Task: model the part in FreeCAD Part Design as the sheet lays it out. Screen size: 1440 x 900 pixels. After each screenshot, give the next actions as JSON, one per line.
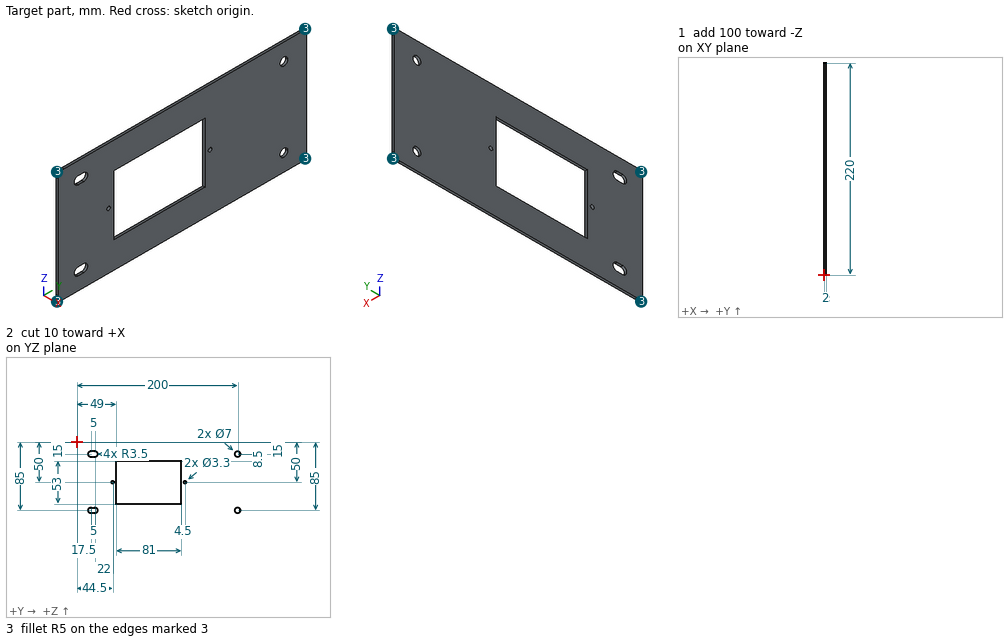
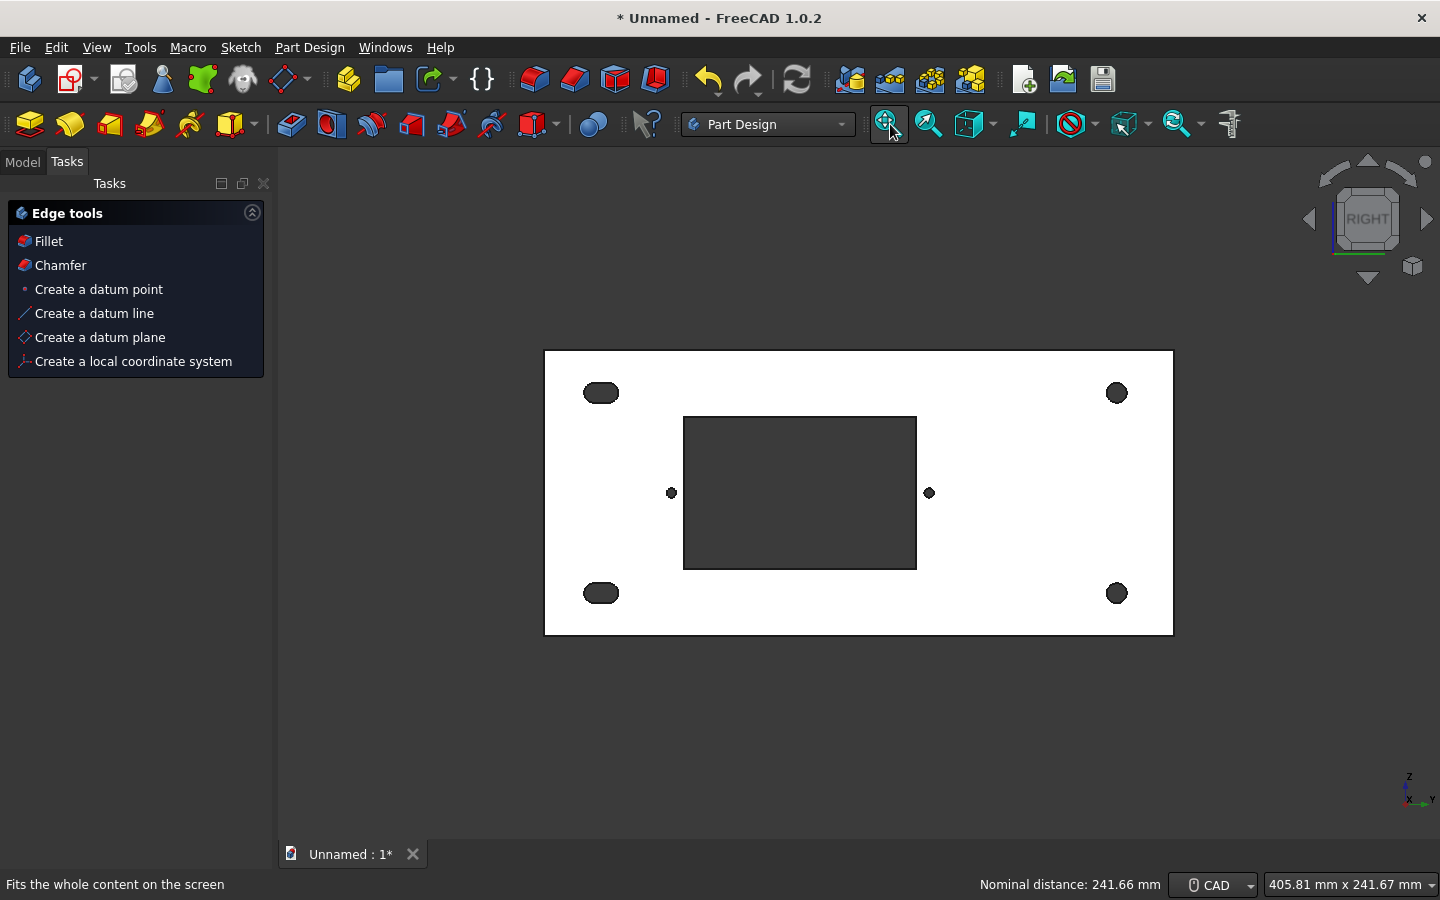
{"action": "key", "text": "5"}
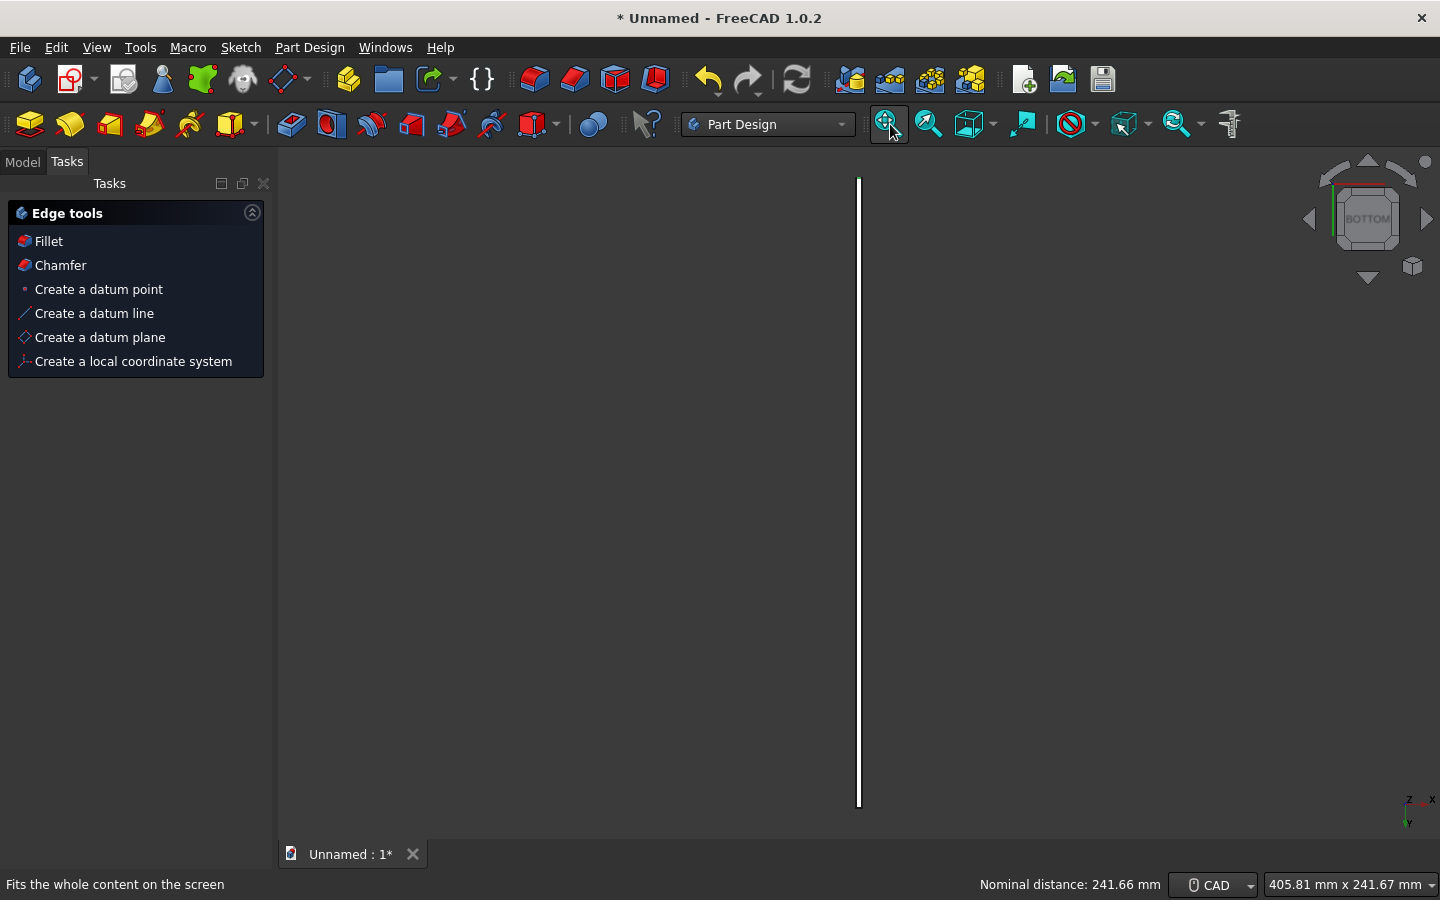
{"action": "scroll", "coordinate": [859, 807], "scroll_direction": "up", "scroll_amount": 10}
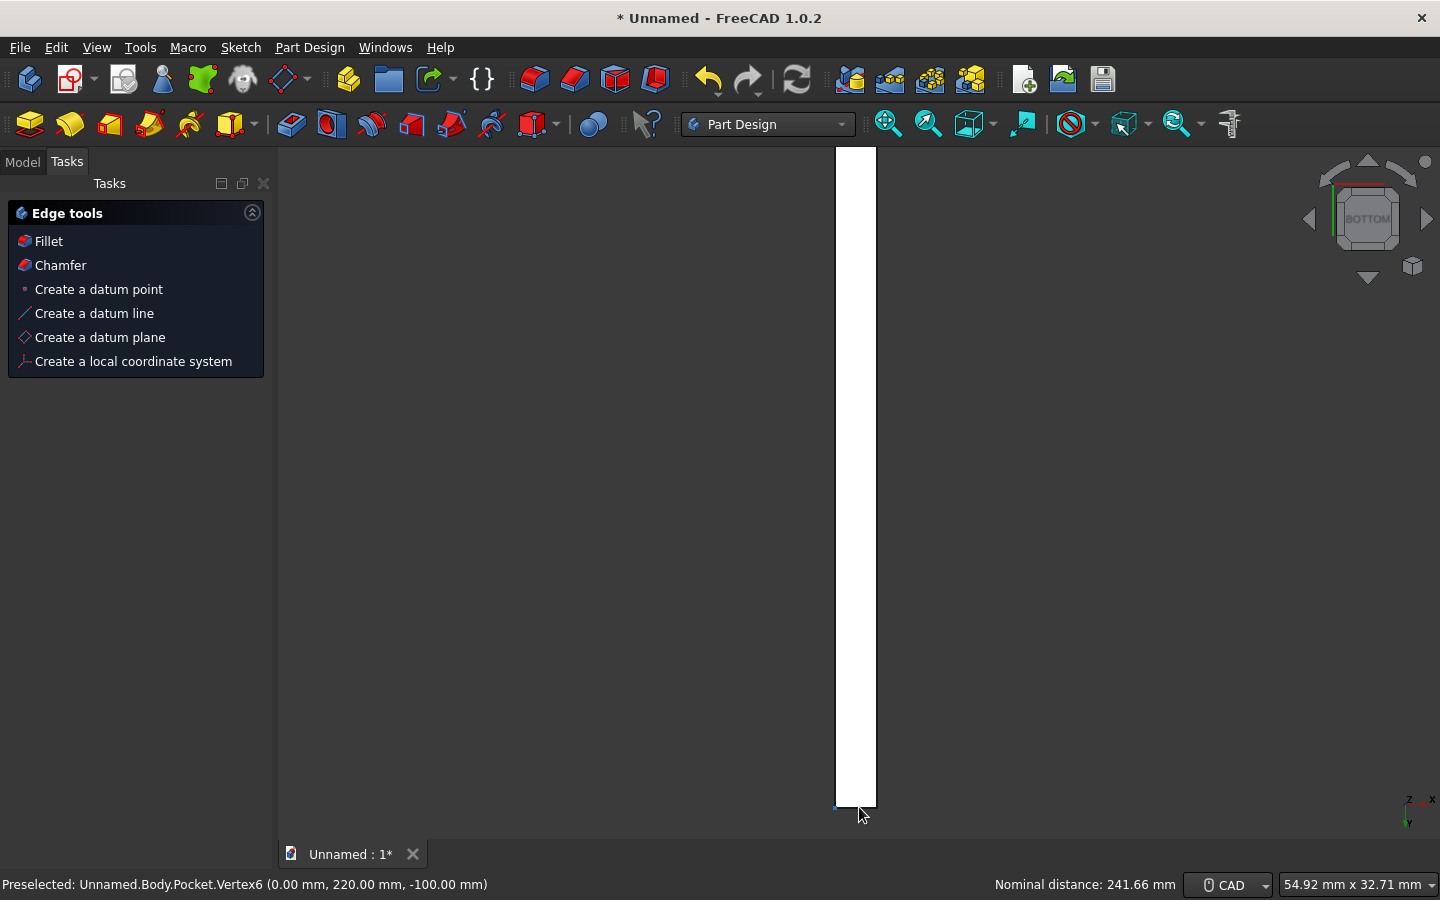
{"action": "left_click", "coordinate": [856, 807], "text": "ctrl"}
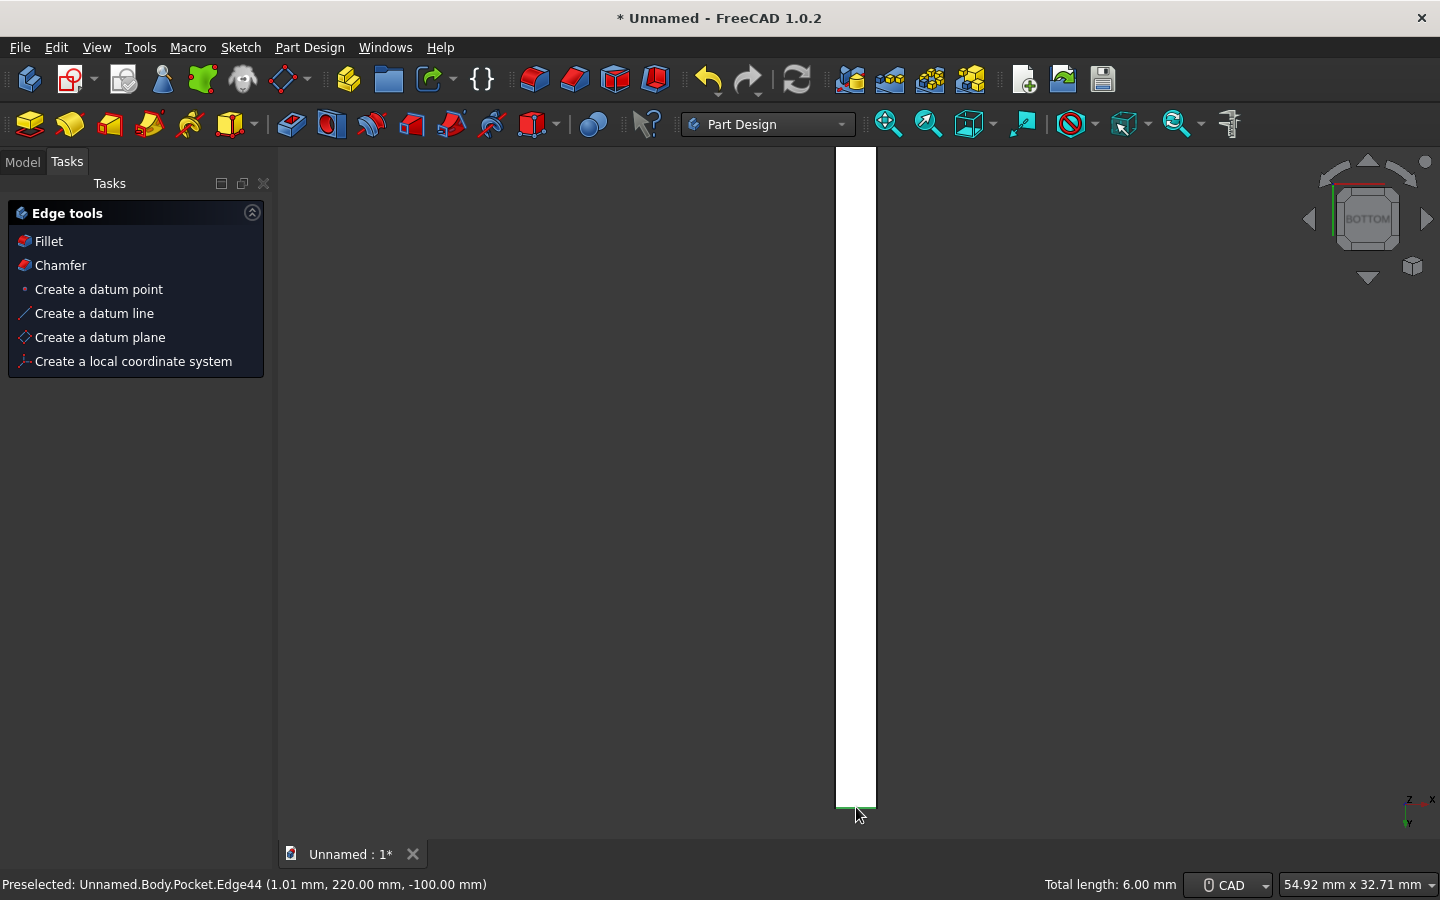
{"action": "left_click", "coordinate": [890, 124]}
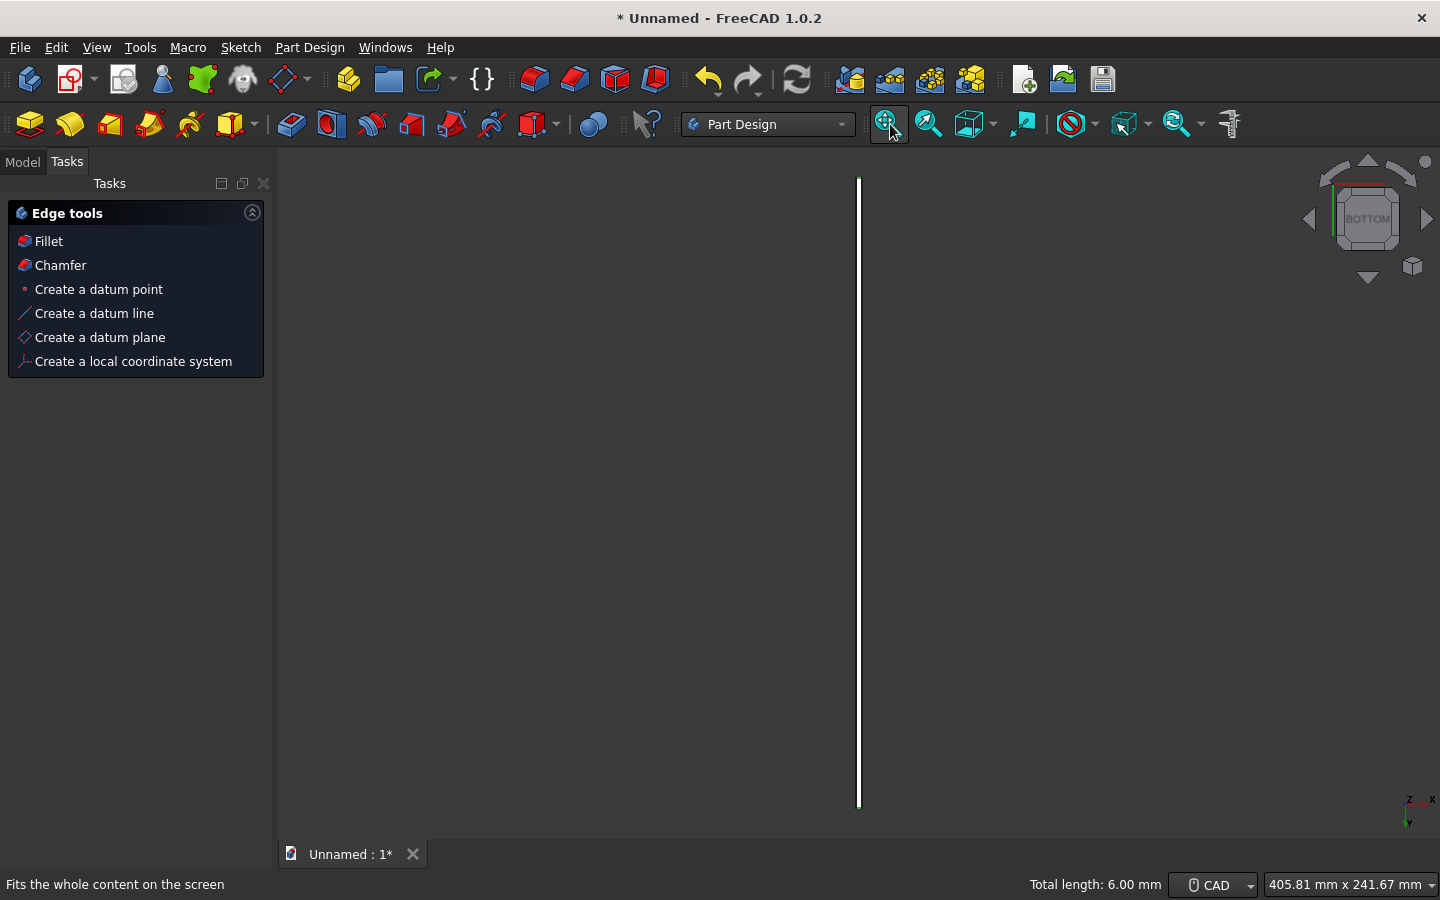
{"action": "key", "text": "4"}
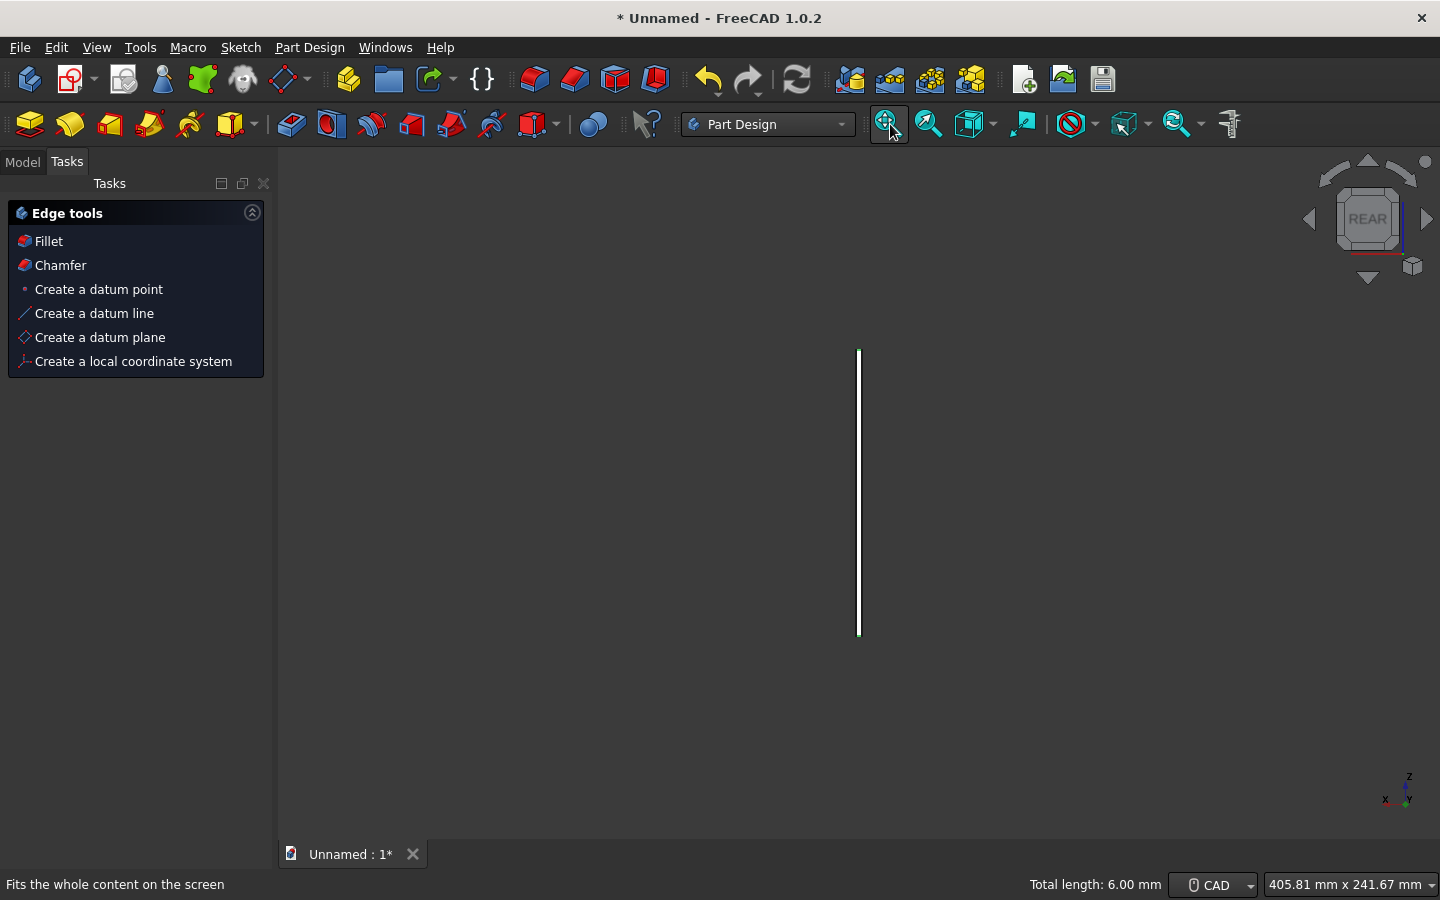
{"action": "left_click", "coordinate": [890, 124]}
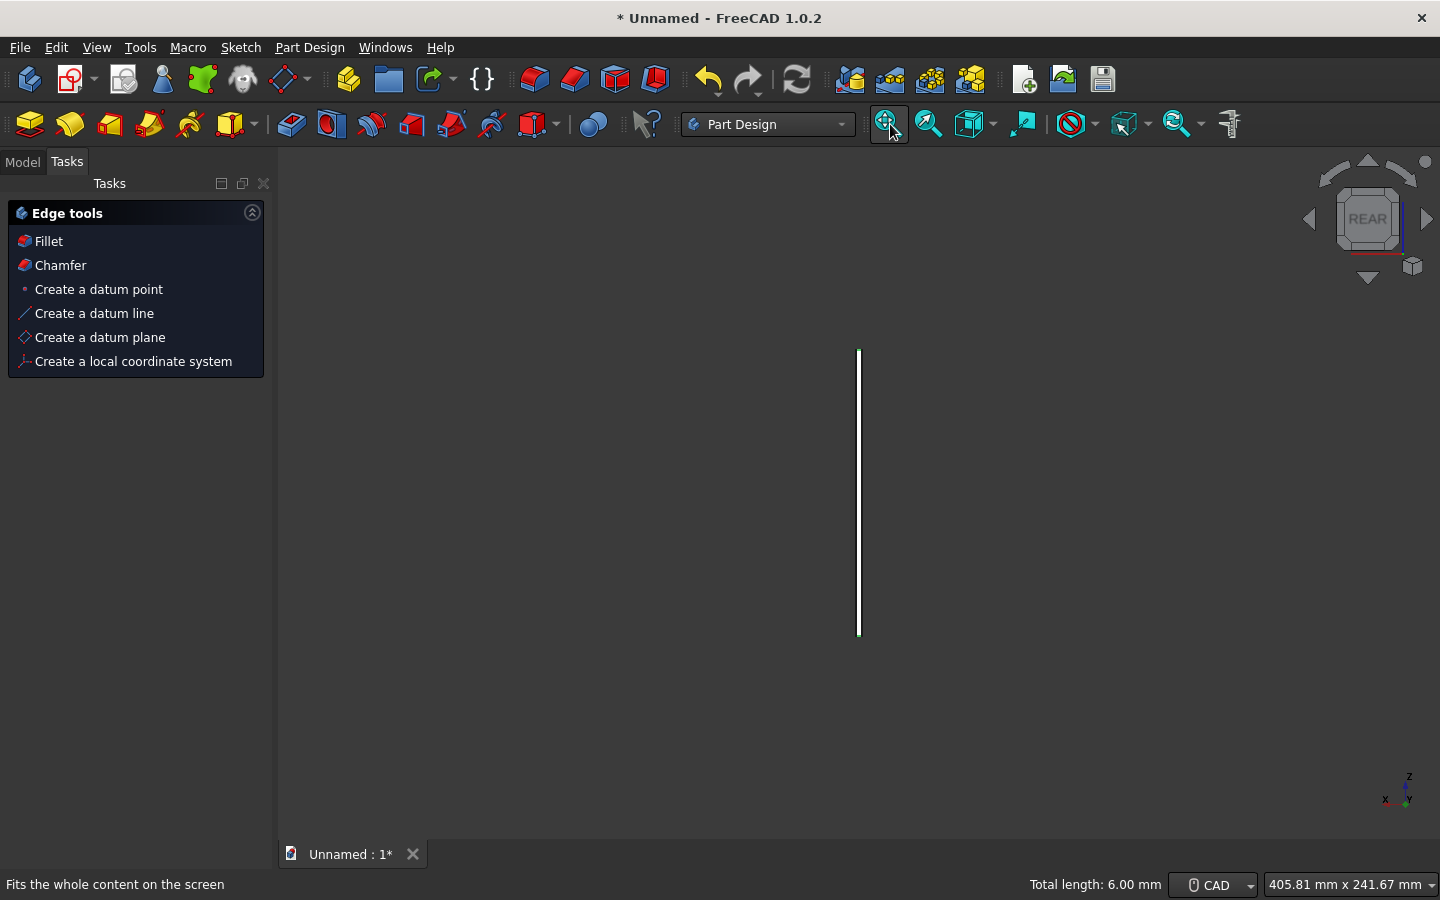
{"action": "scroll", "coordinate": [859, 349], "scroll_direction": "up", "scroll_amount": 10}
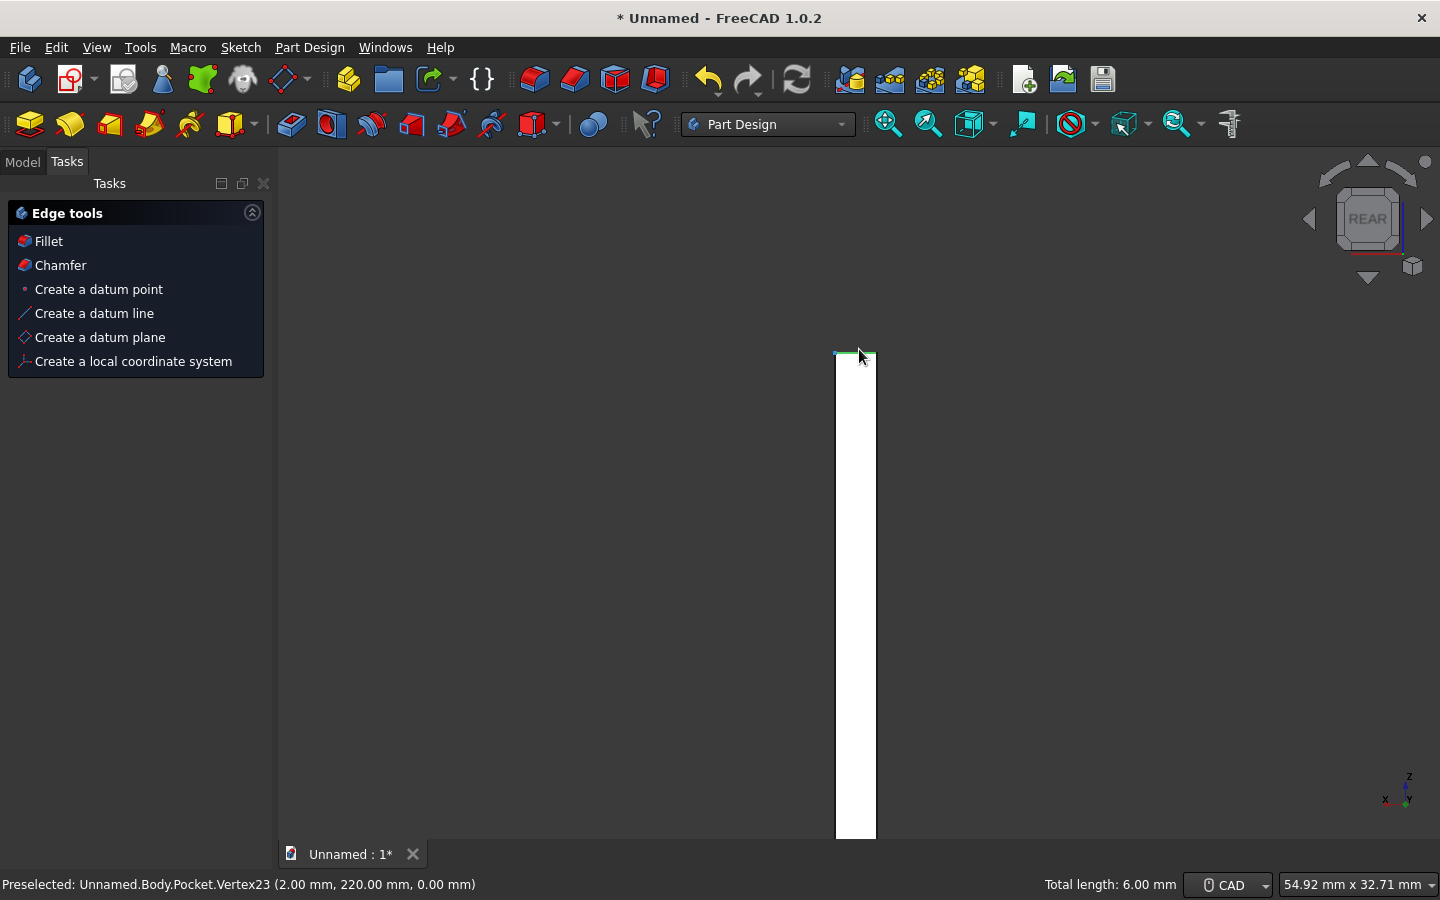
{"action": "left_click", "coordinate": [890, 124]}